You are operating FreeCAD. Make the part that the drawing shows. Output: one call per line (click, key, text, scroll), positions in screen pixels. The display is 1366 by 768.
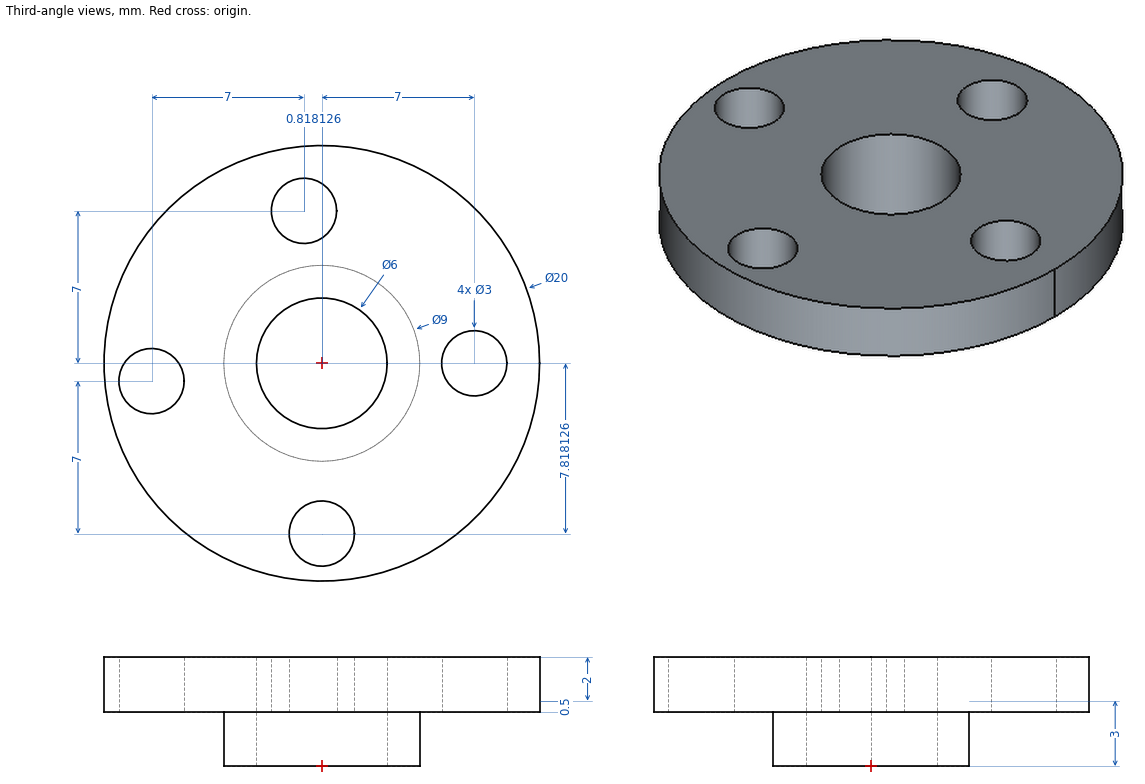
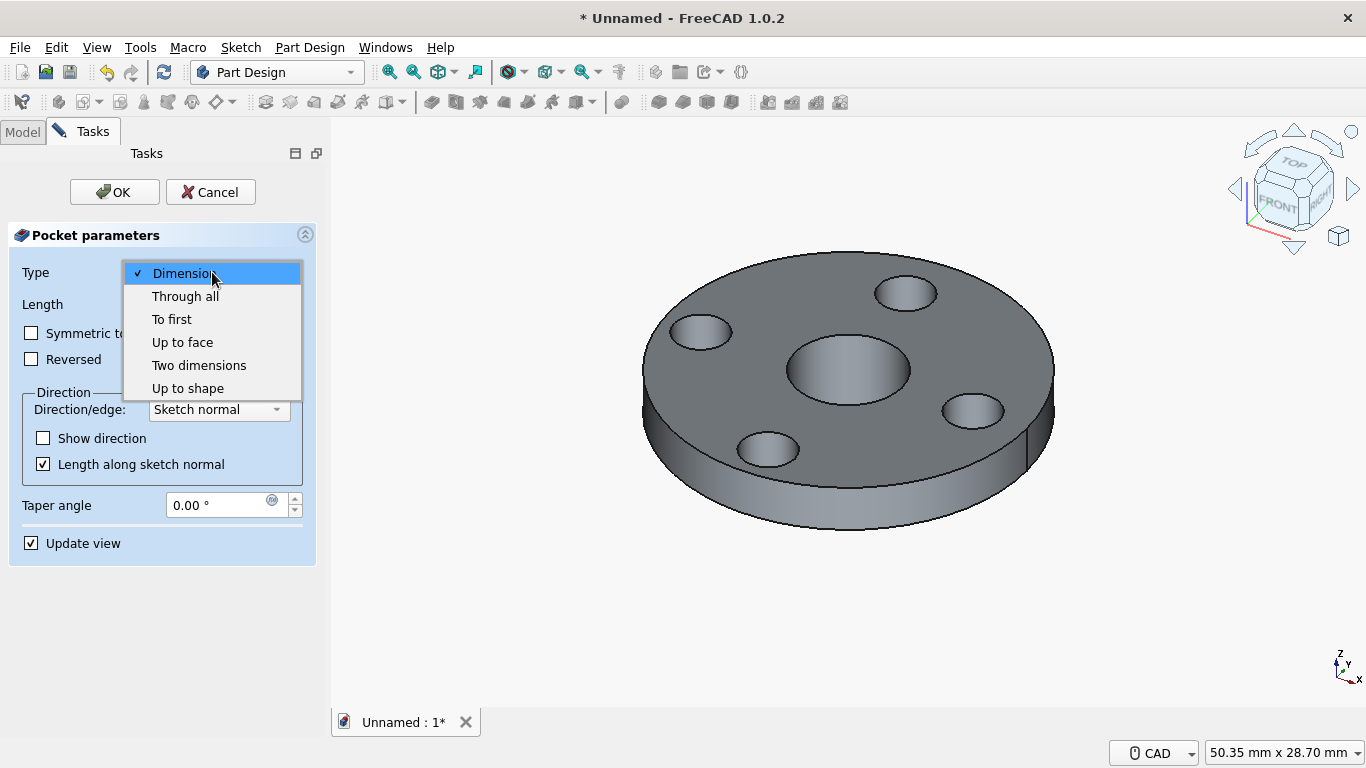
click(212, 296)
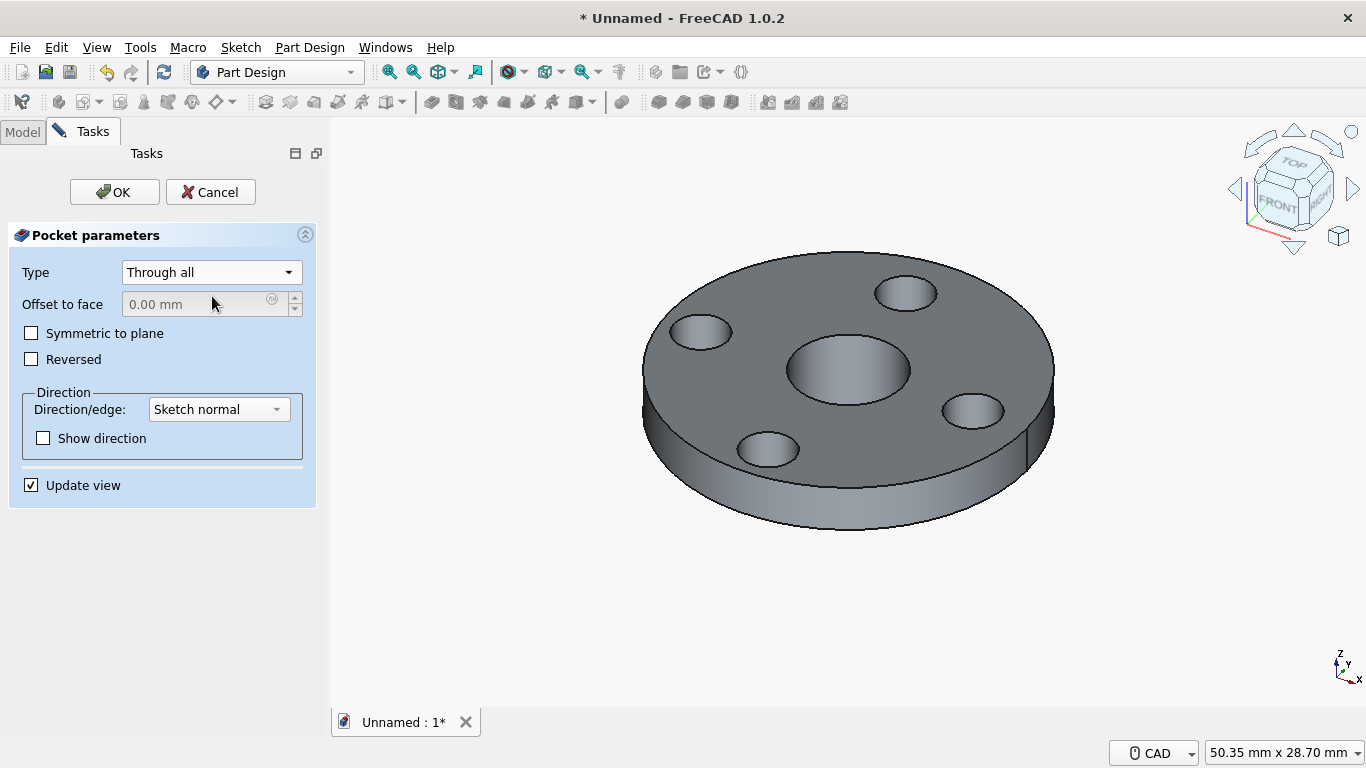
click(115, 192)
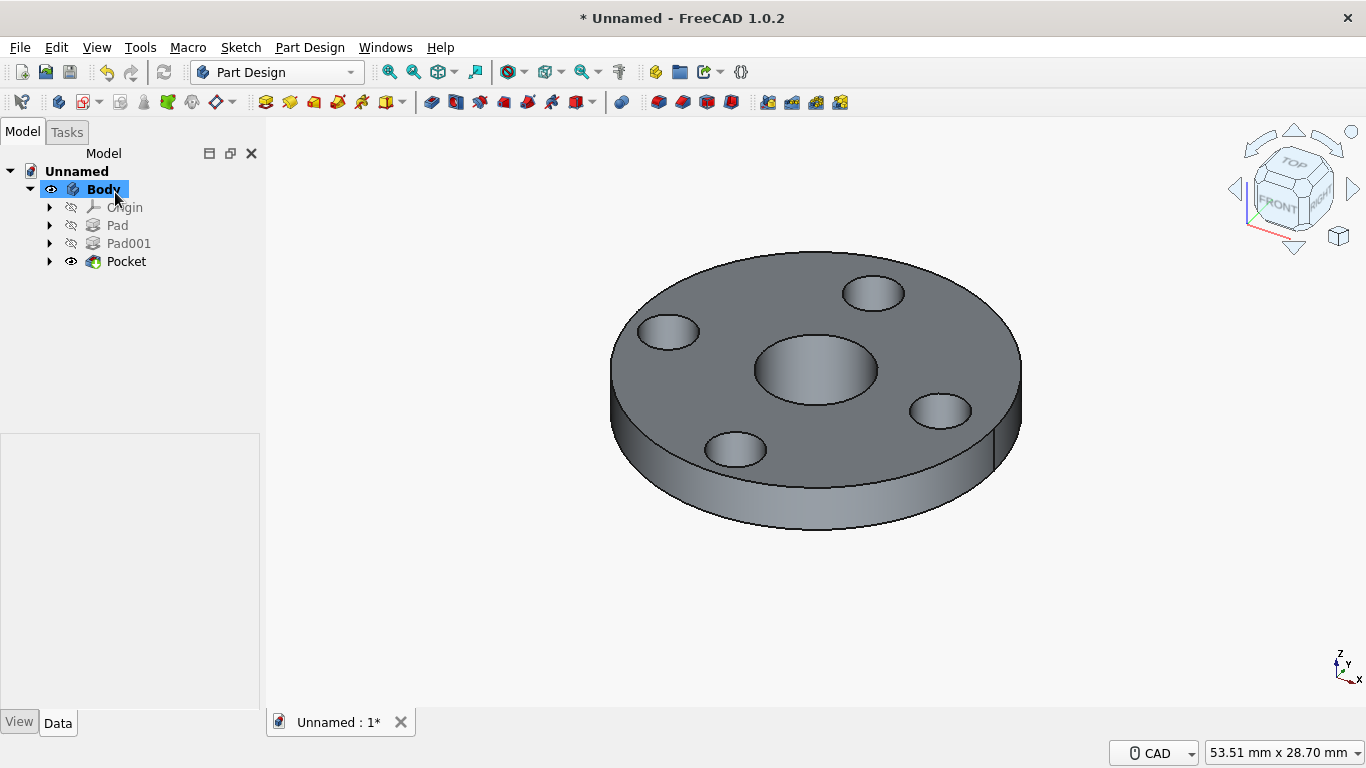
key(0)